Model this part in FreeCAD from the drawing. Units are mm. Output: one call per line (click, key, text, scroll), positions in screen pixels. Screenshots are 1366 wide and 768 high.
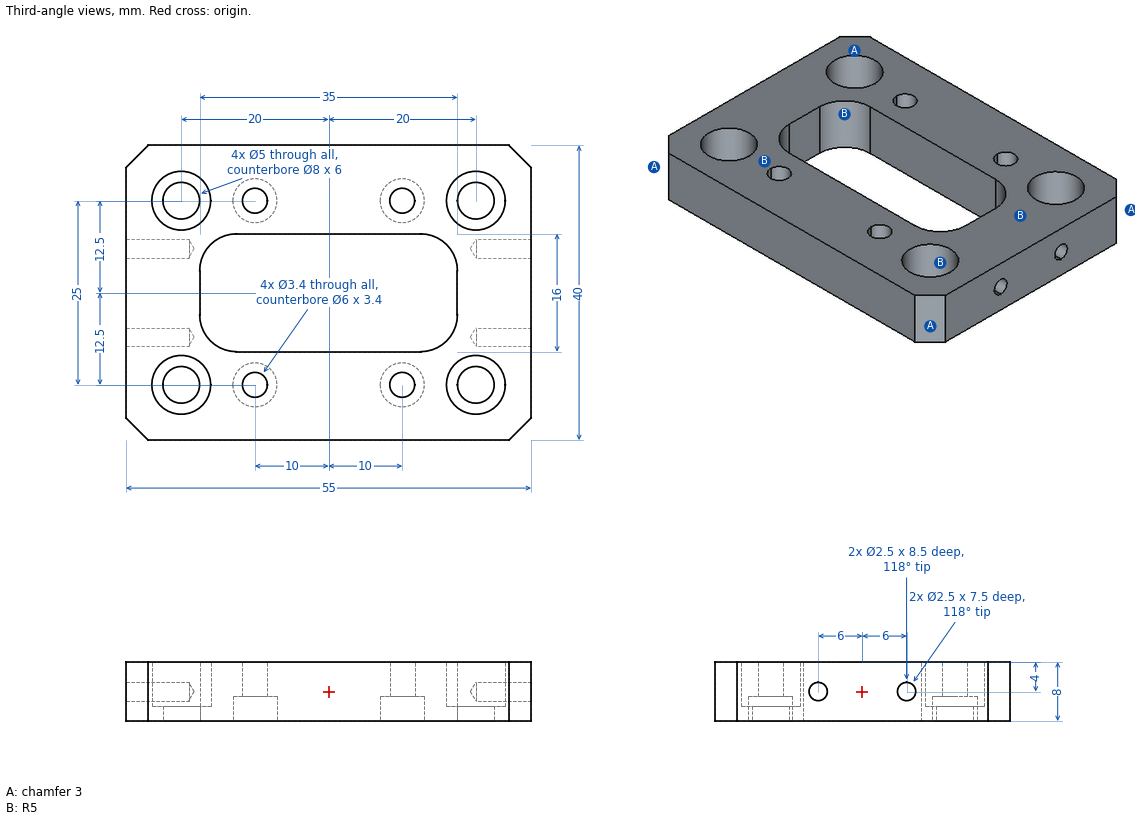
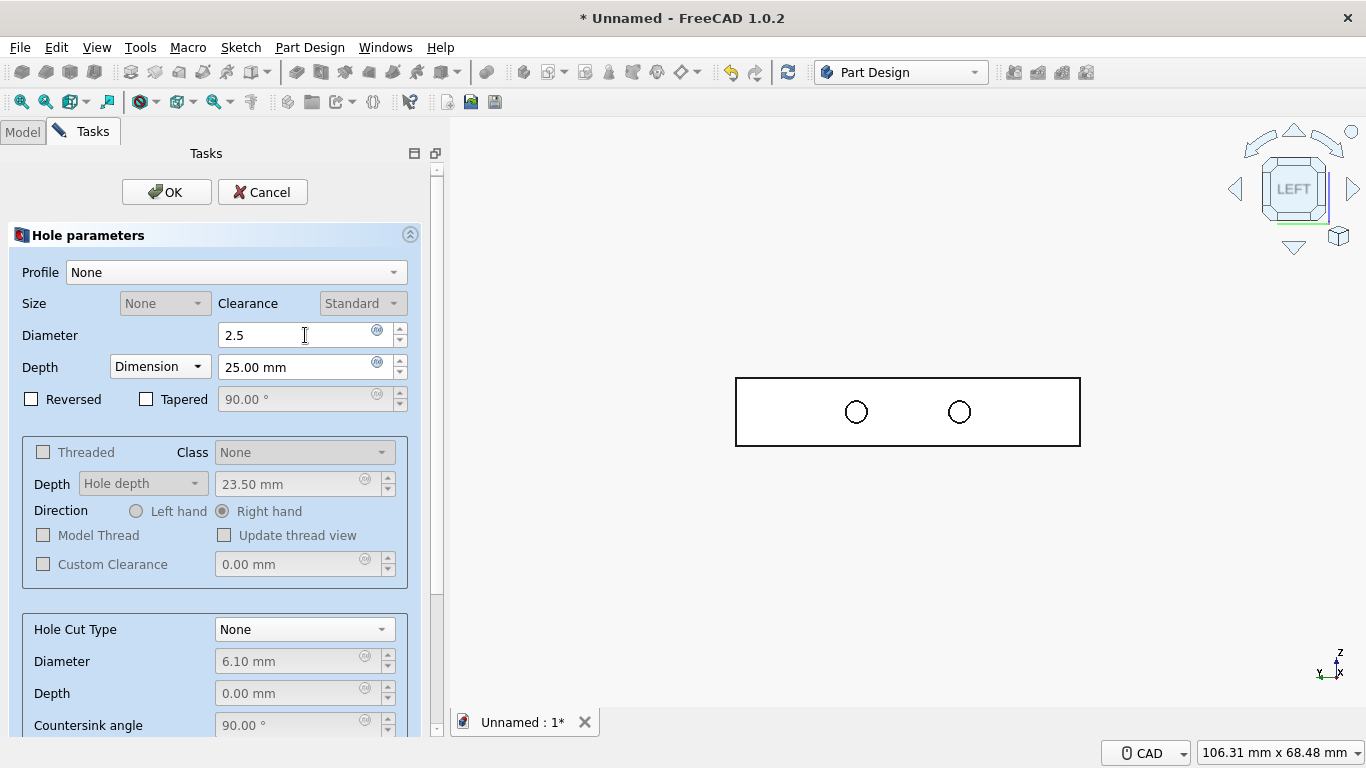
triple_click(305, 367)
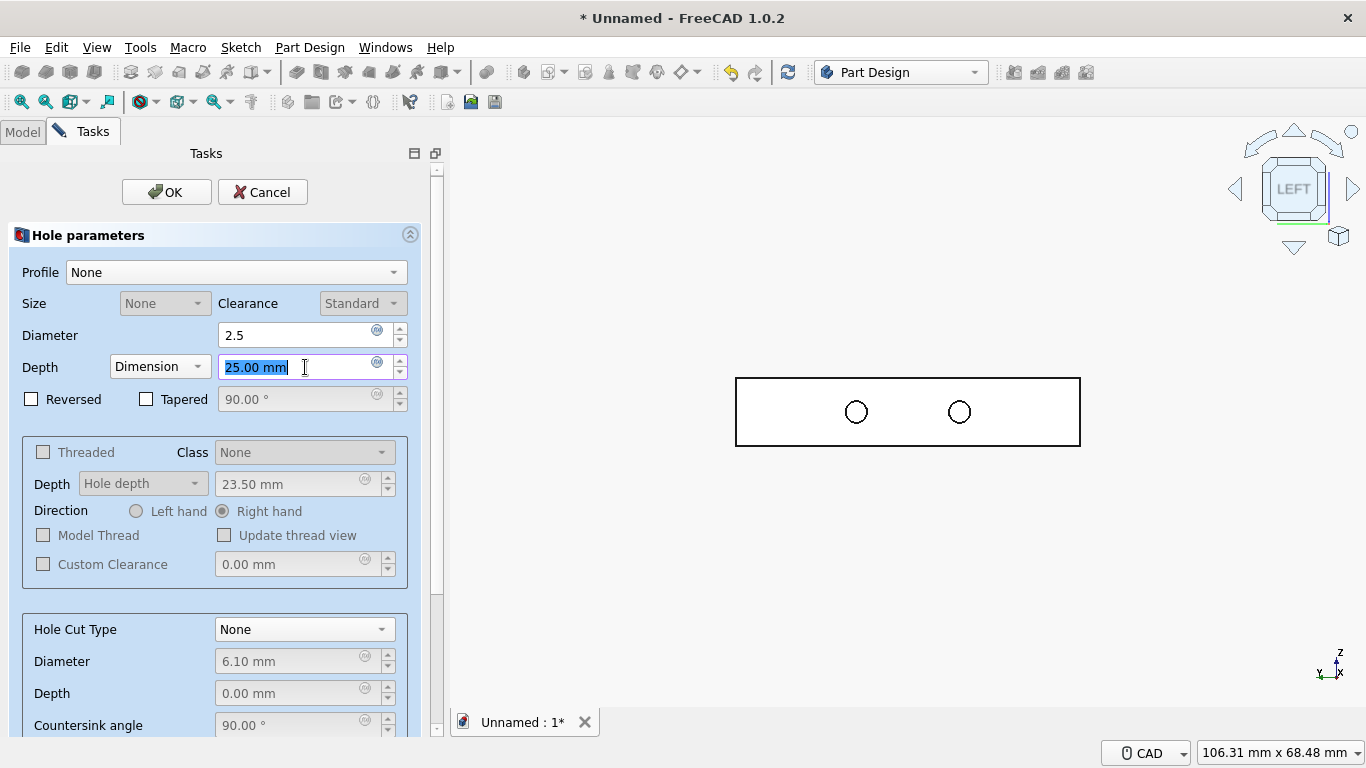
text(8.5)
key(Tab)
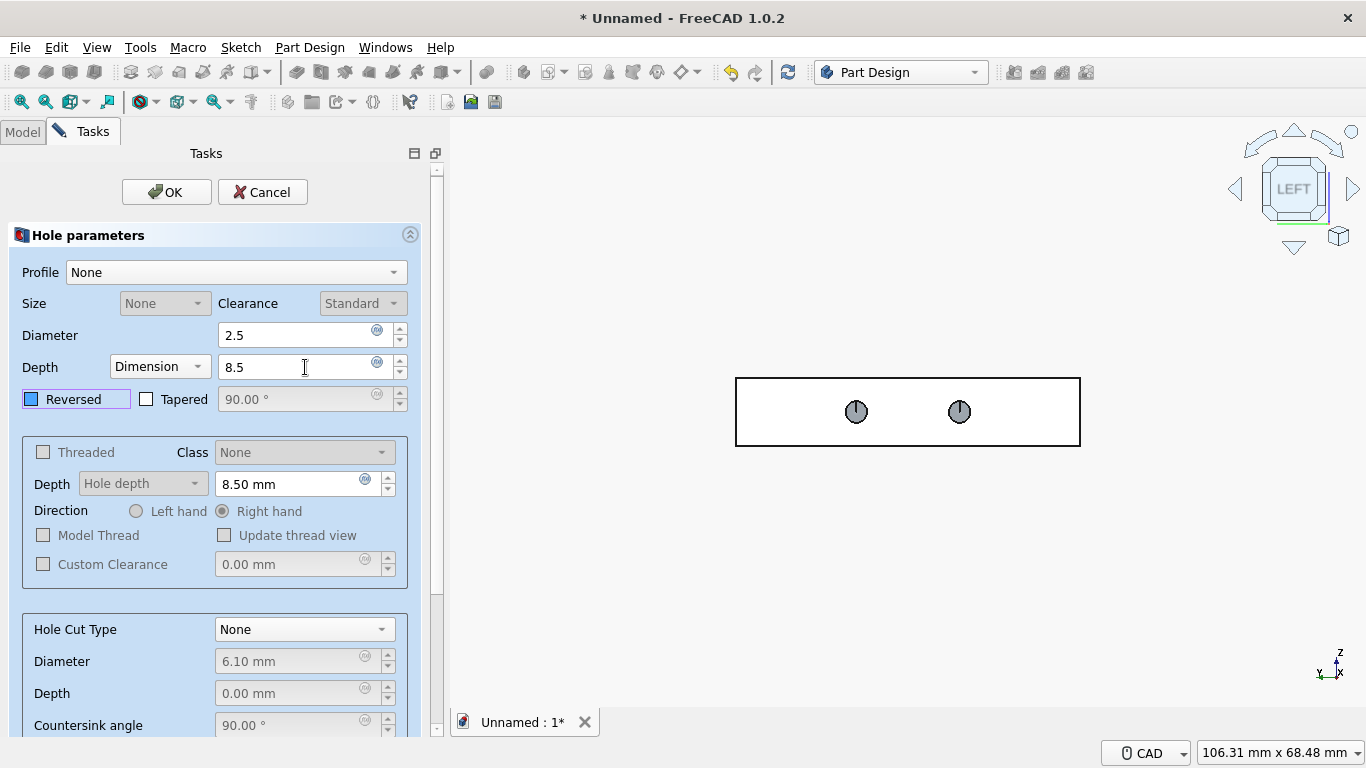
click(167, 192)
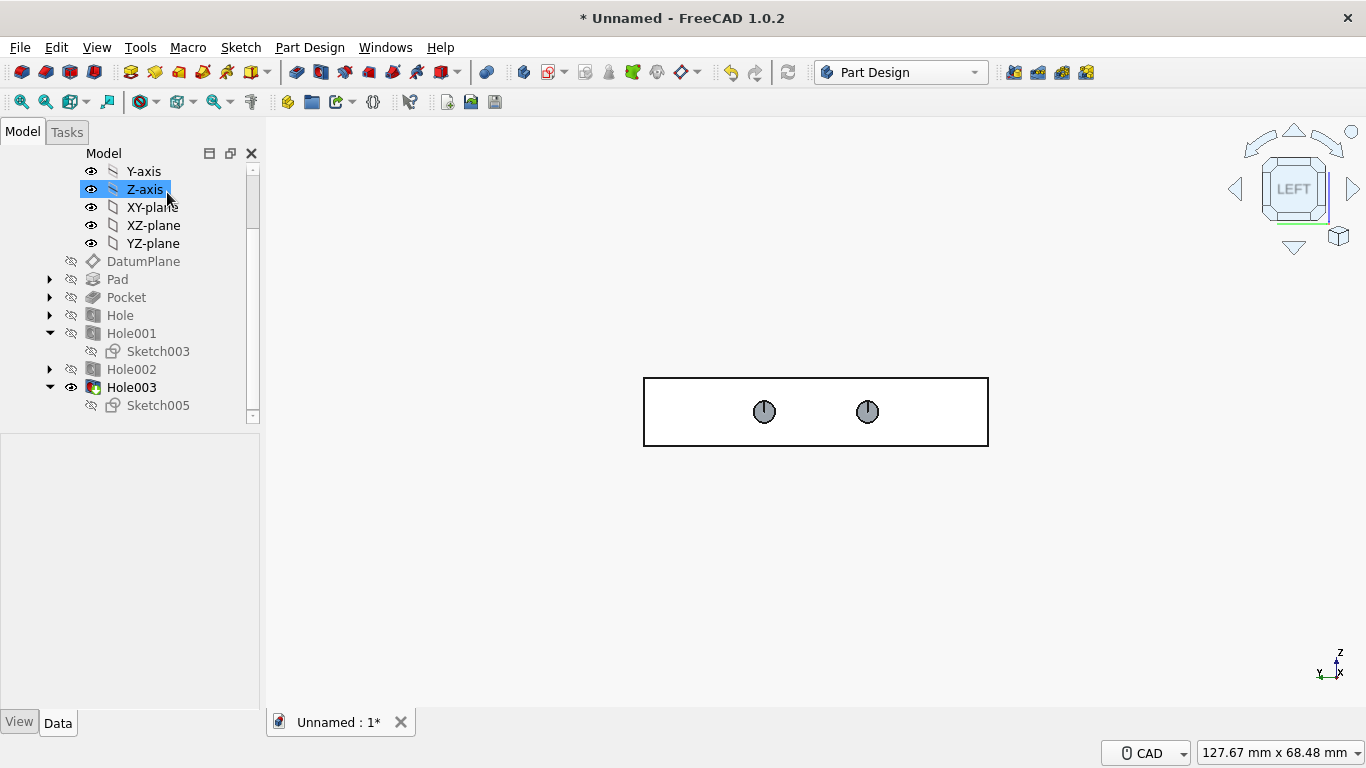
click(22, 102)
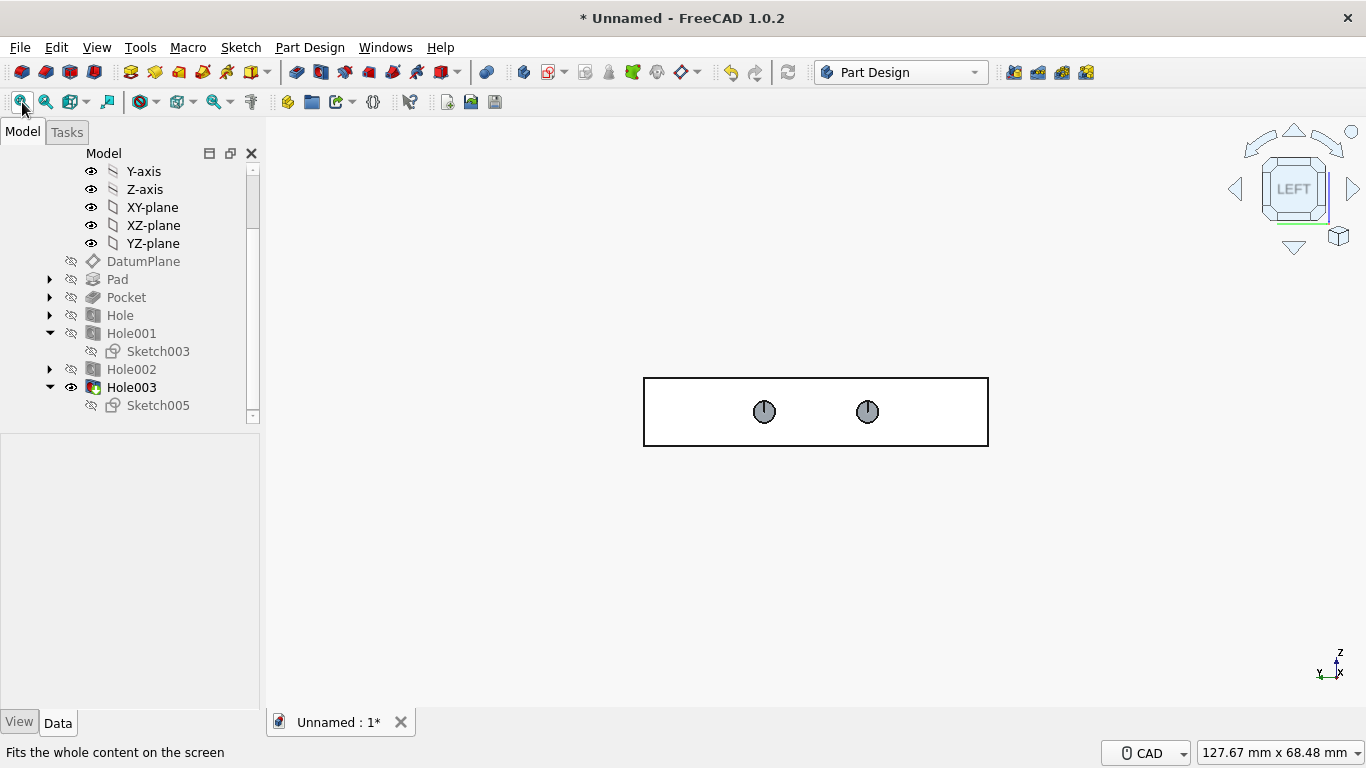
click(988, 411)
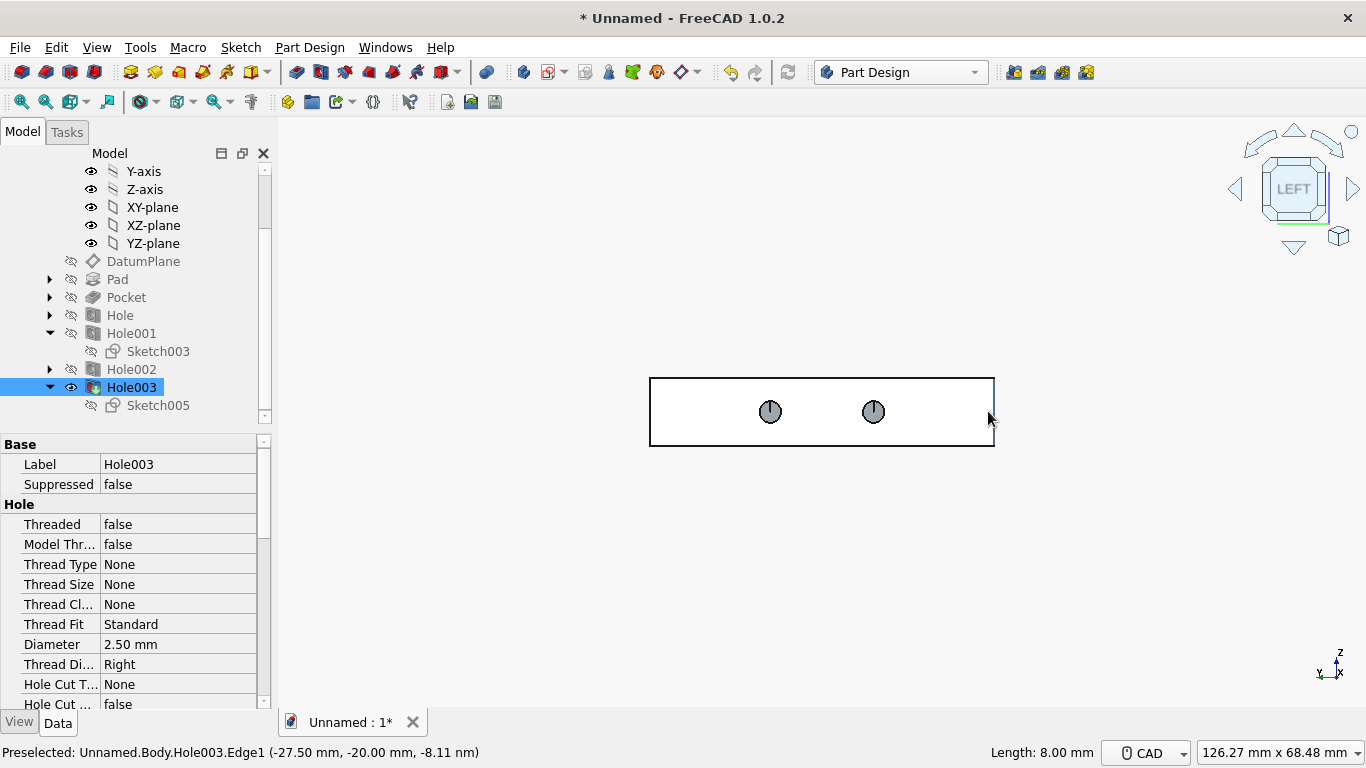
click(650, 411, ctrl)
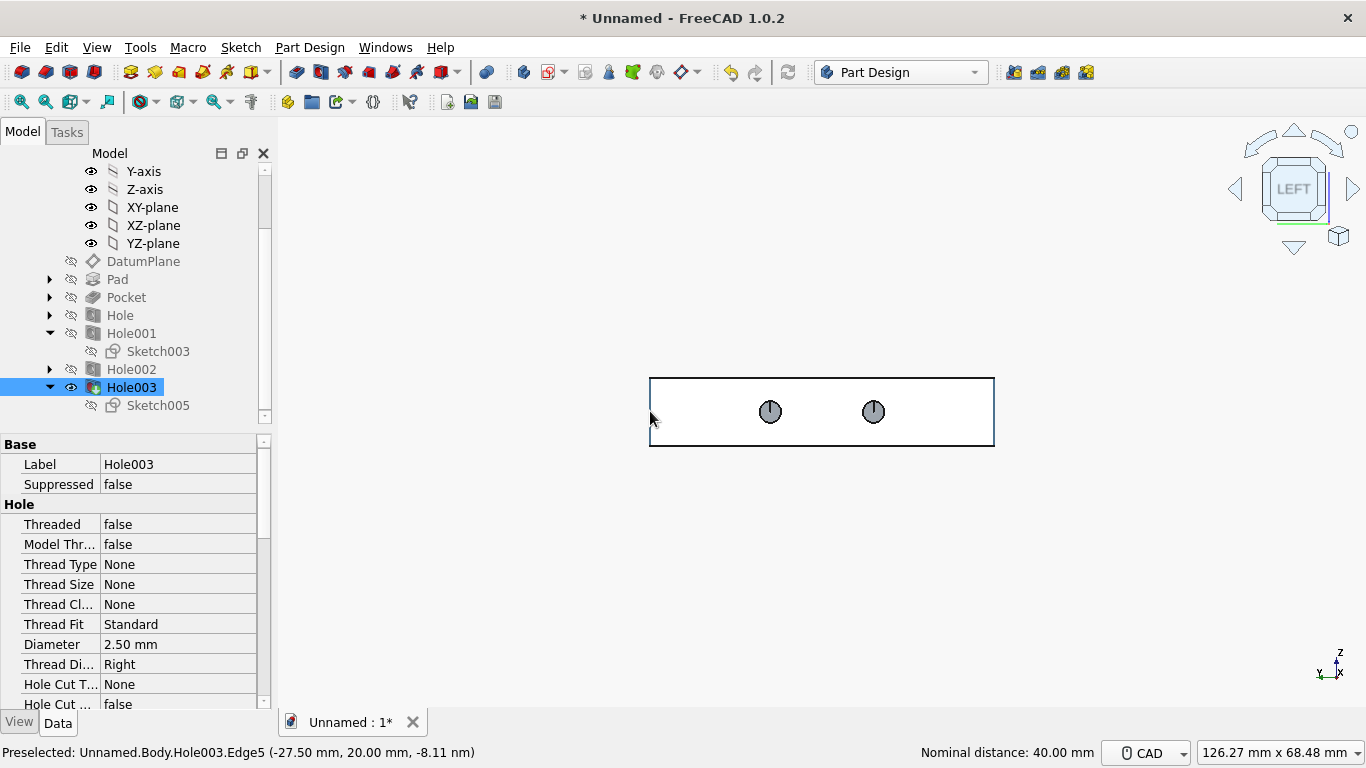
key(0)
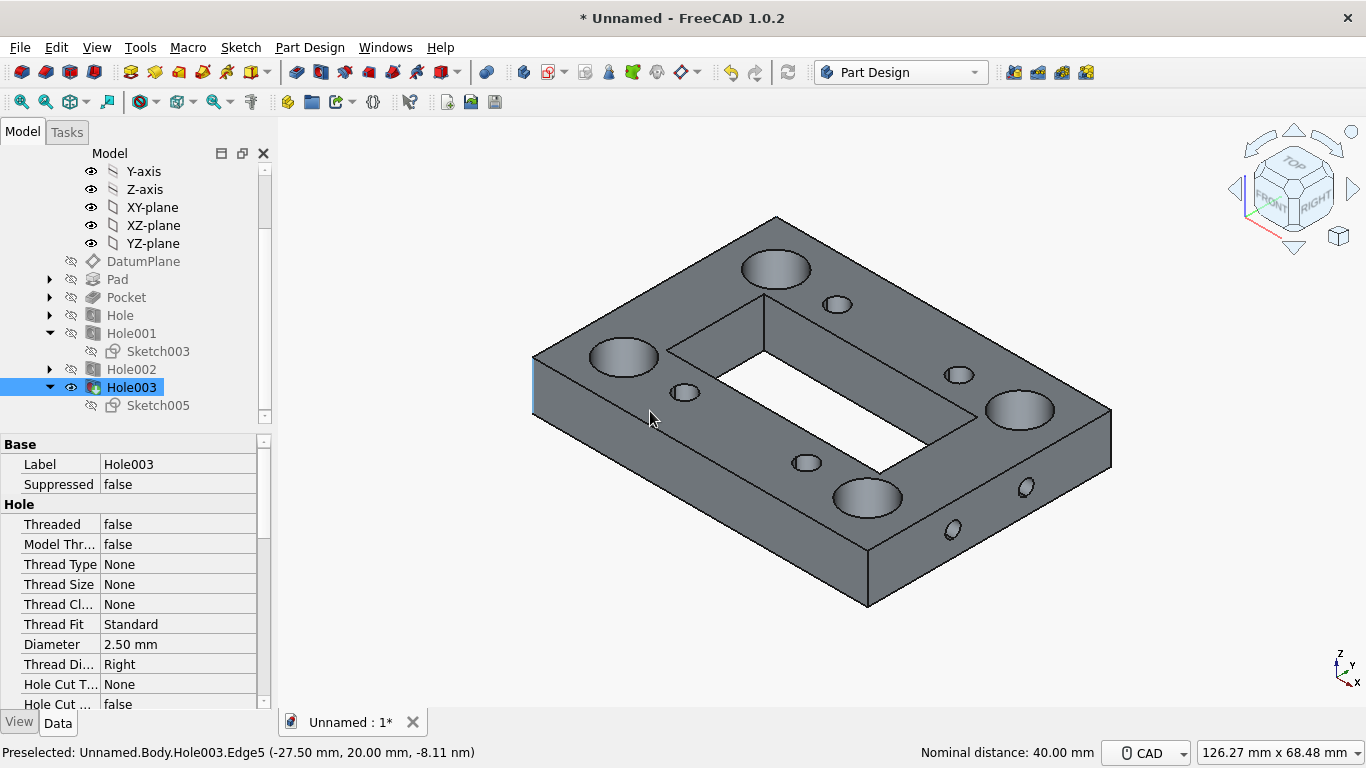
click(868, 578, ctrl)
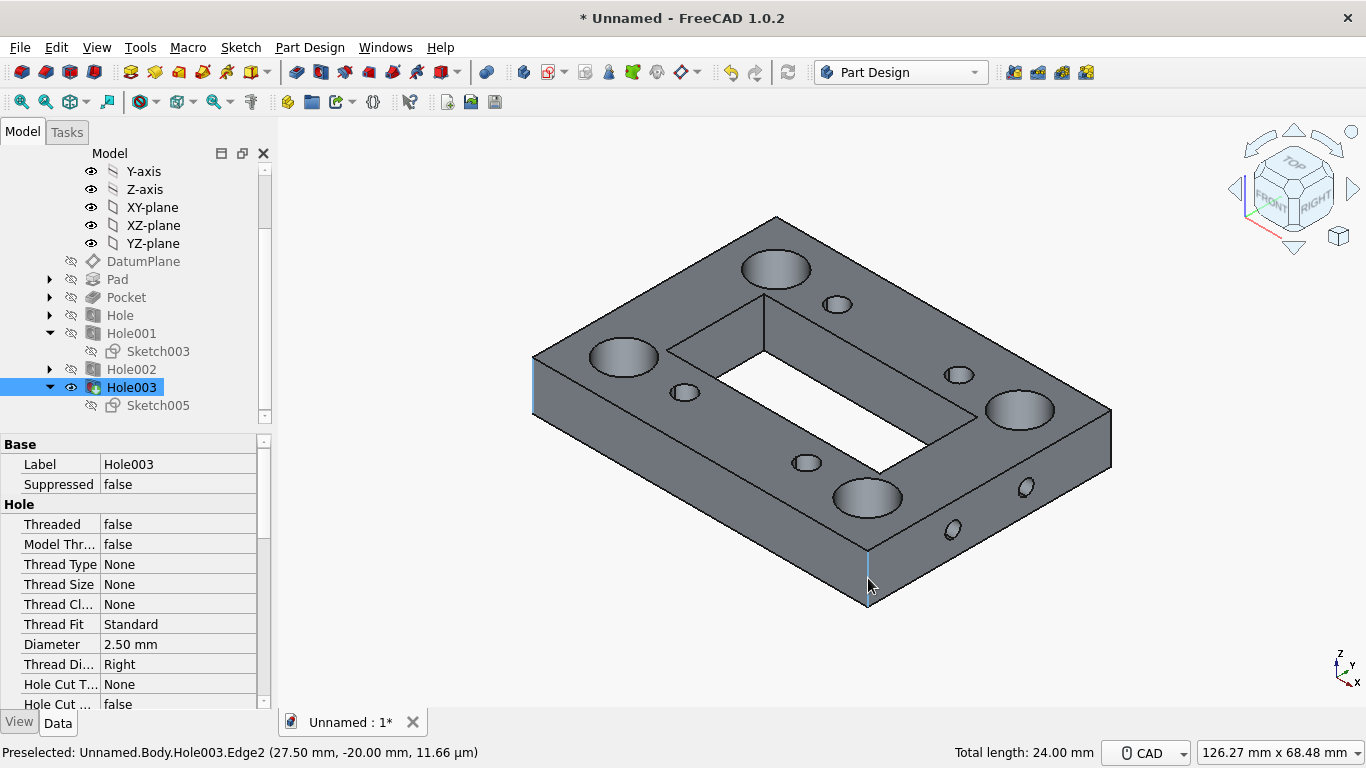
key(2)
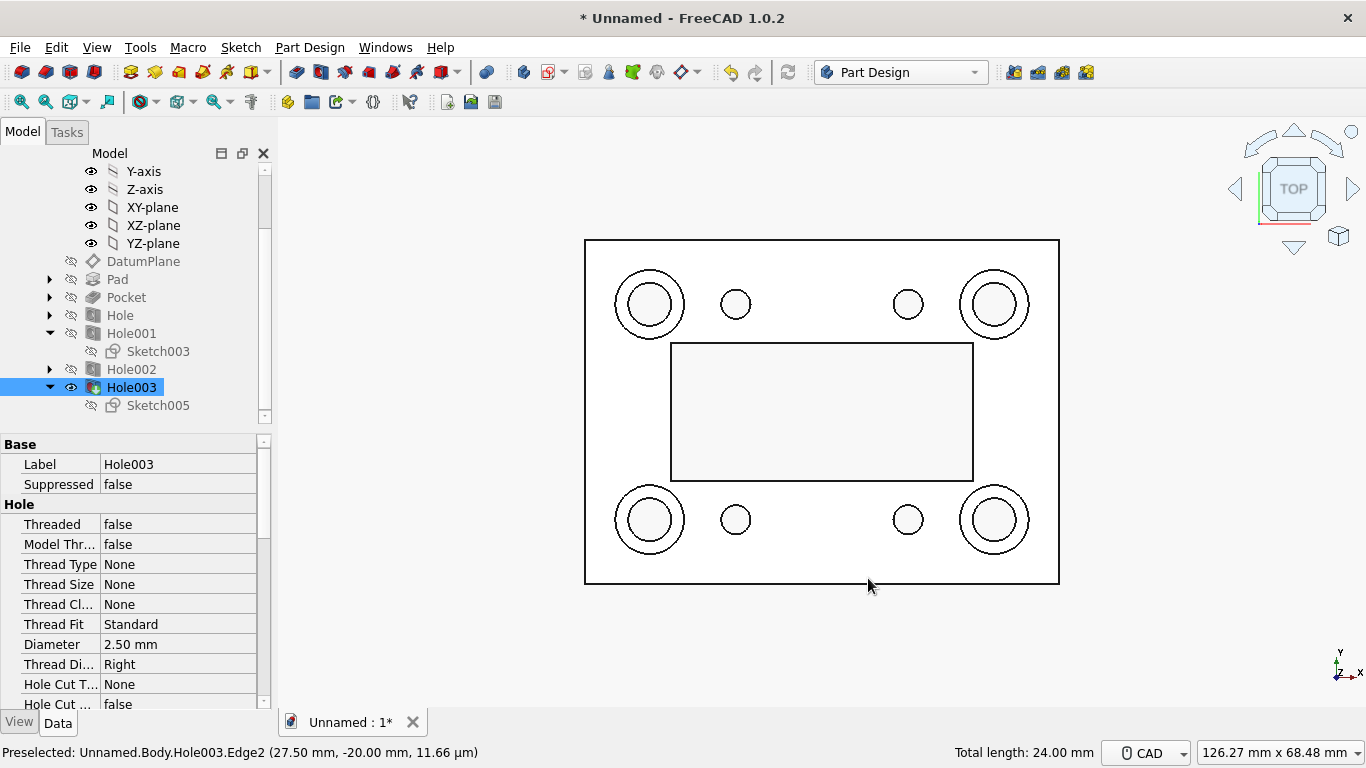
key(1)